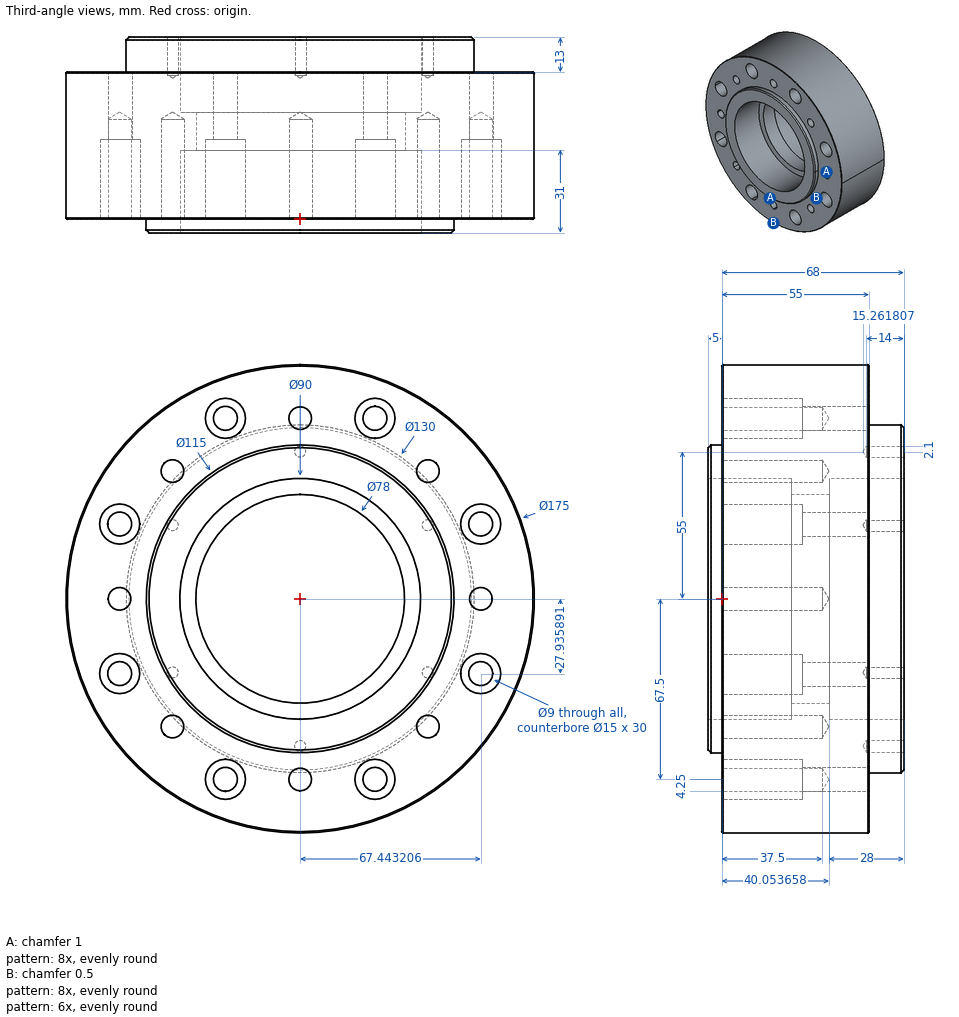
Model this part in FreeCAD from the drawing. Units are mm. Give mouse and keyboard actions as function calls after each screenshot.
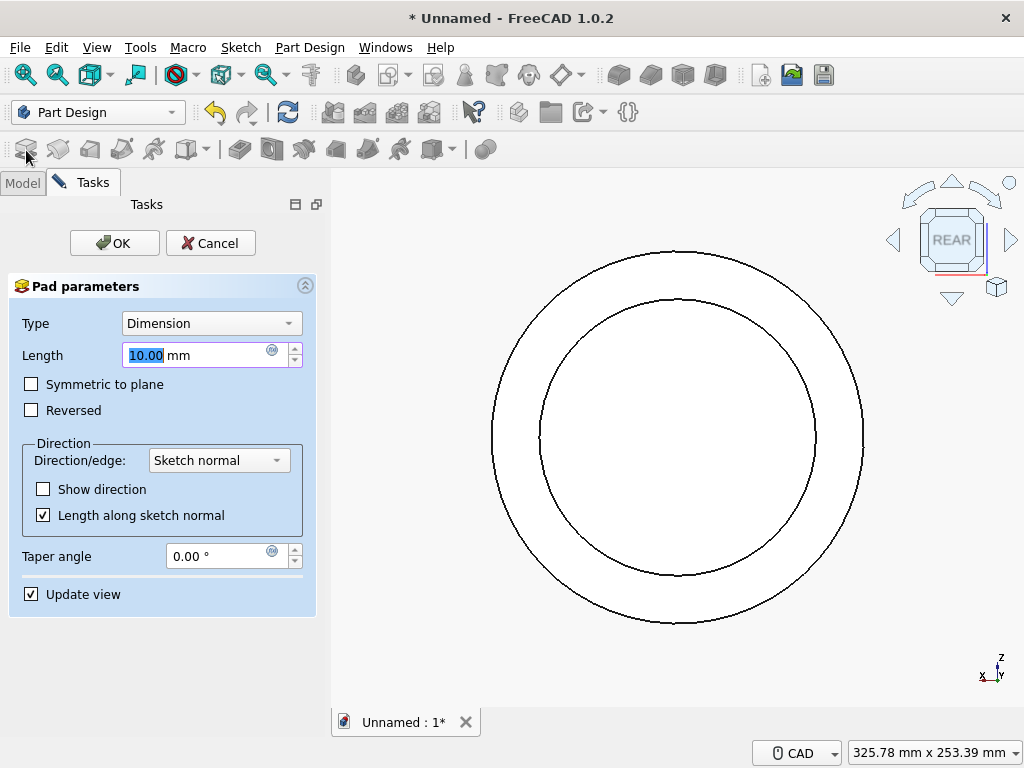
text(5)
key(Tab)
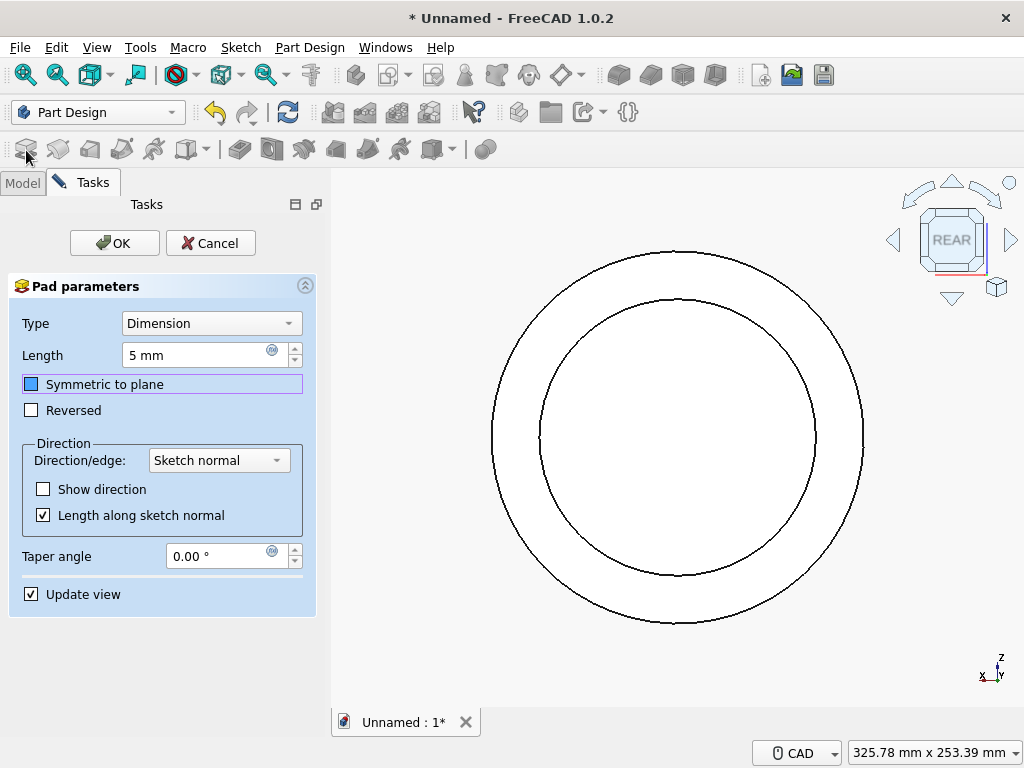
click(115, 243)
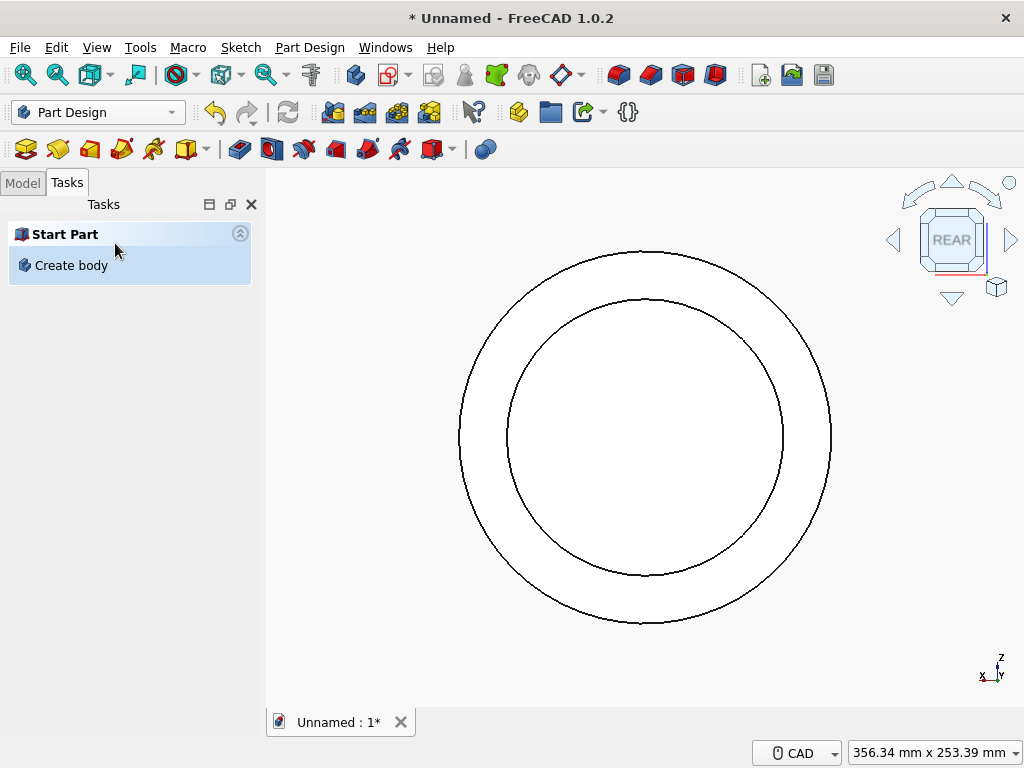
key(0)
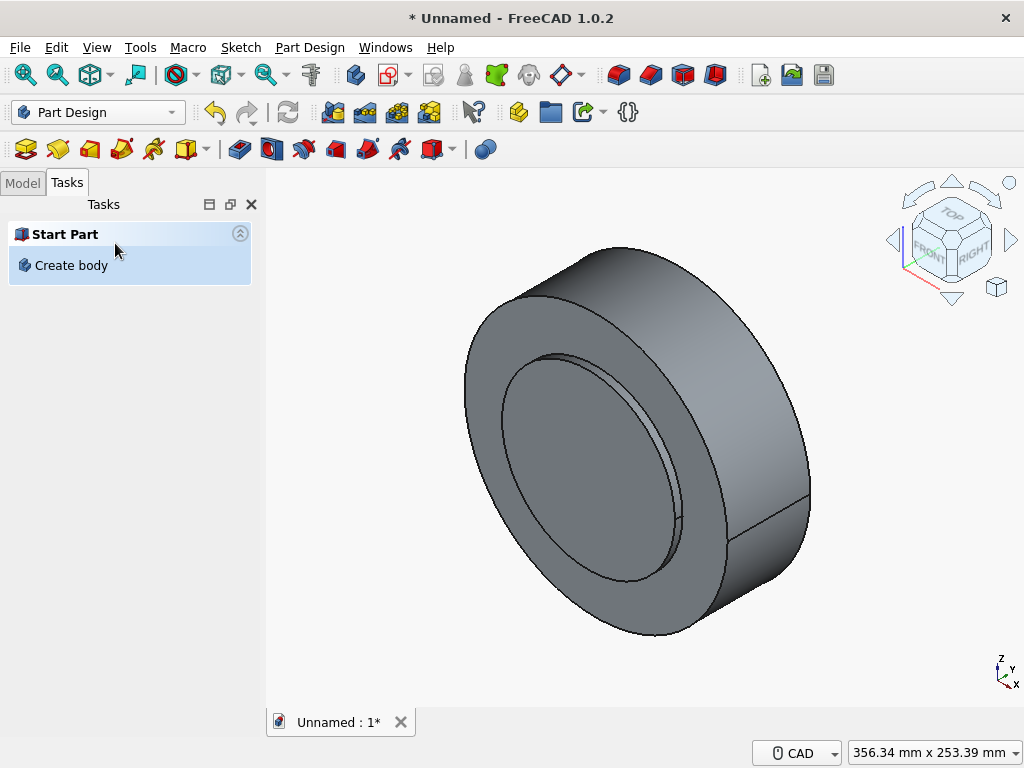
click(588, 469)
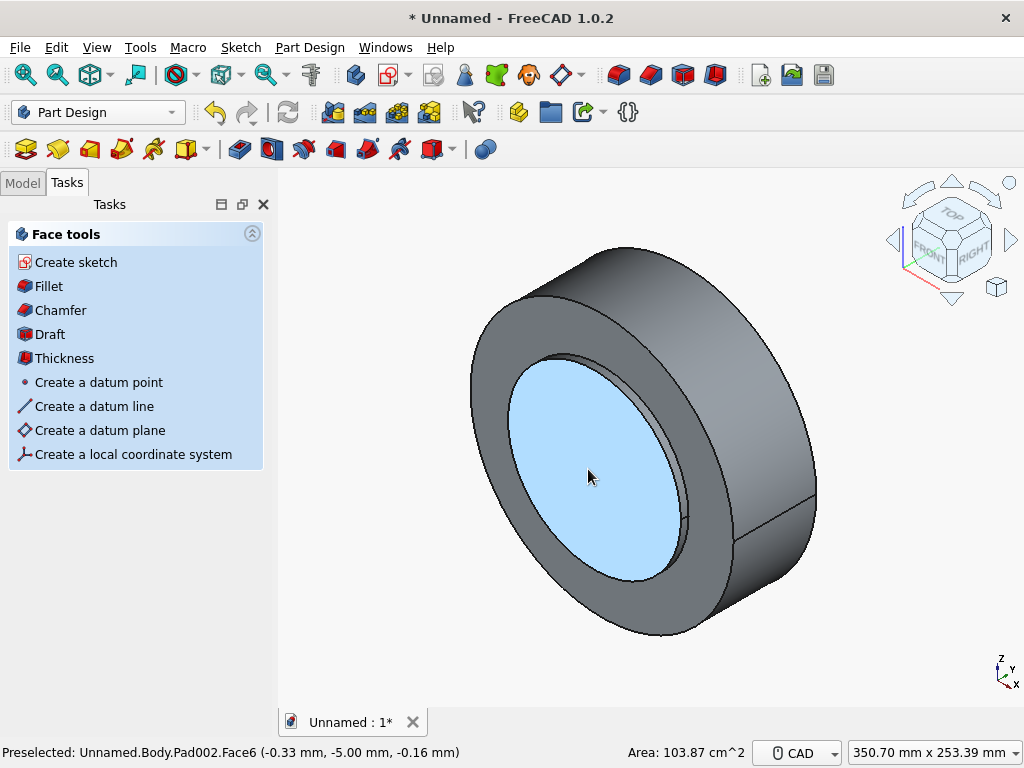
click(388, 76)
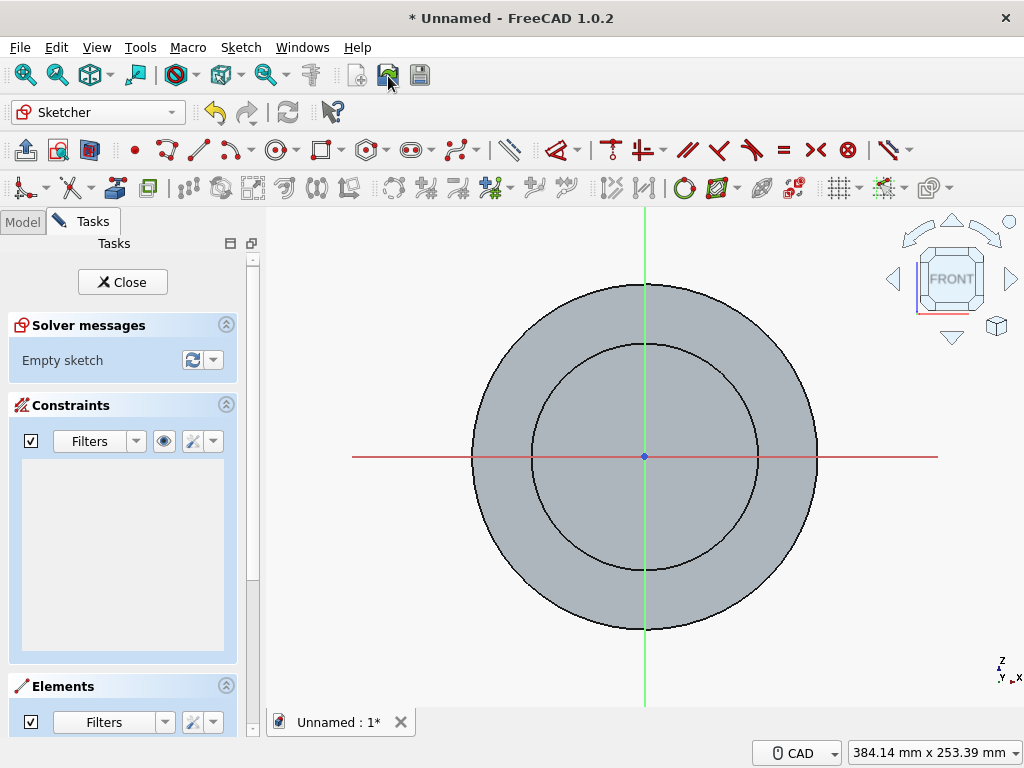
scroll(728, 457, up, 3)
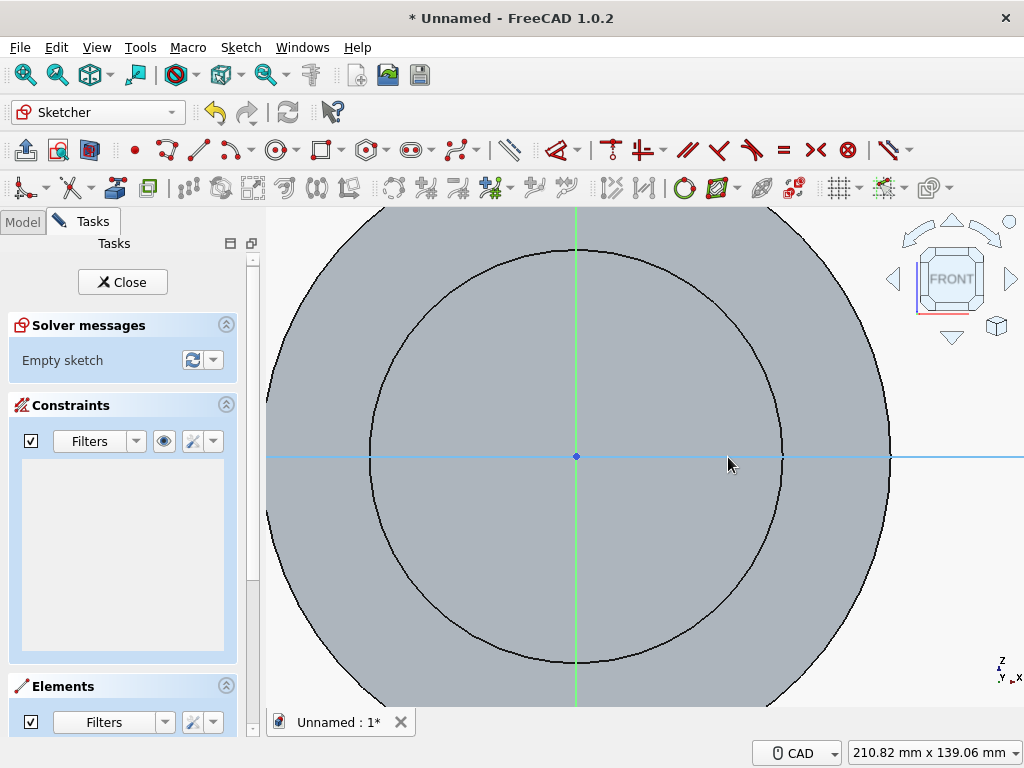
click(276, 150)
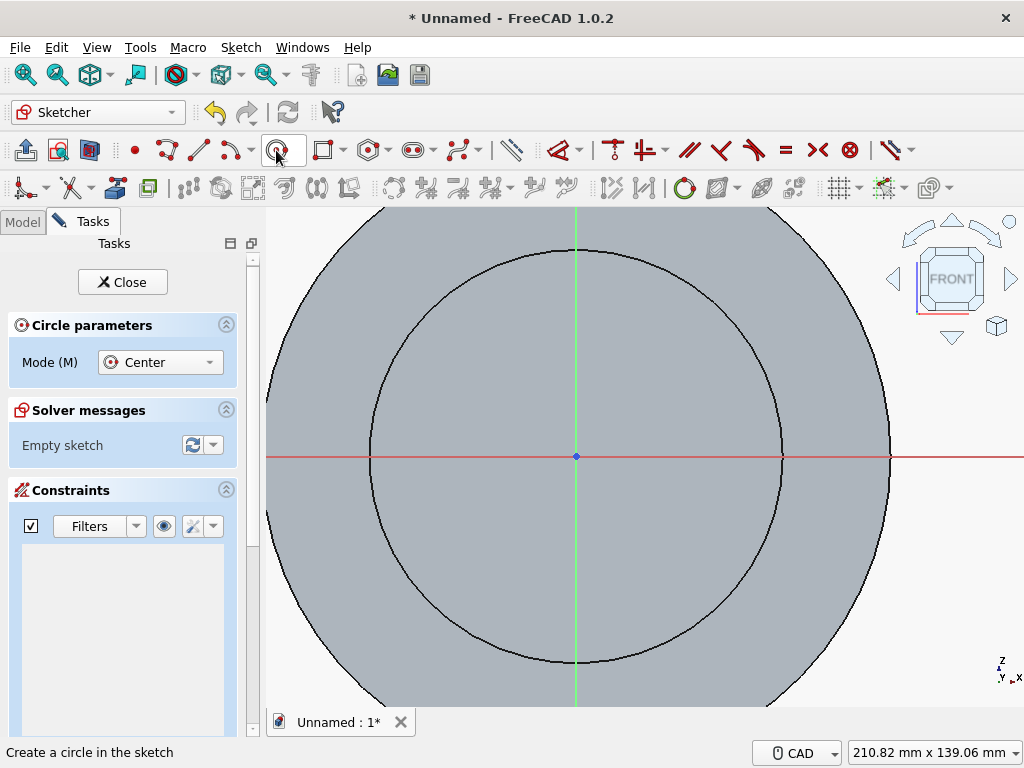
click(576, 457)
click(690, 342)
key(Escape)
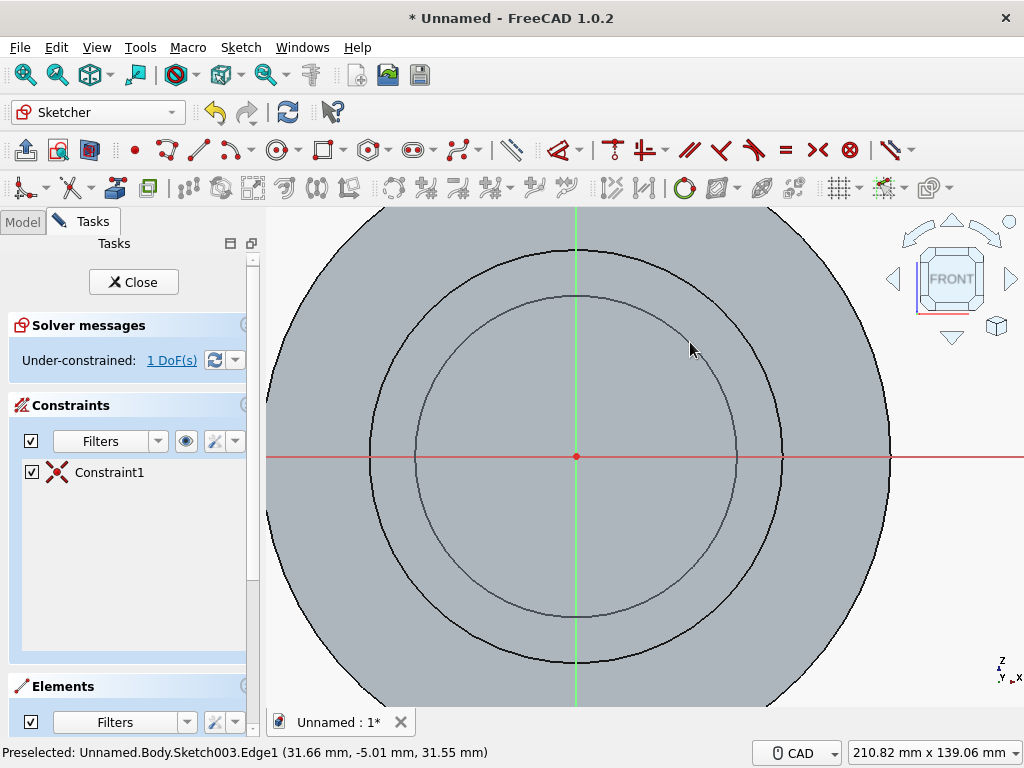
click(558, 150)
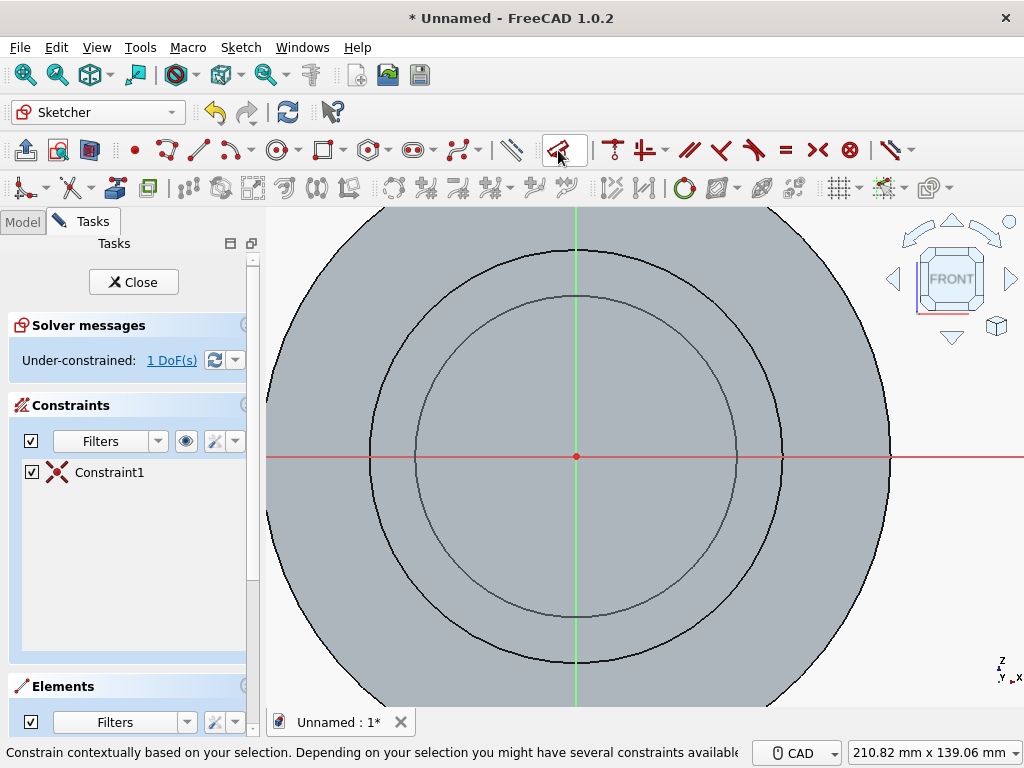
click(689, 342)
click(711, 319)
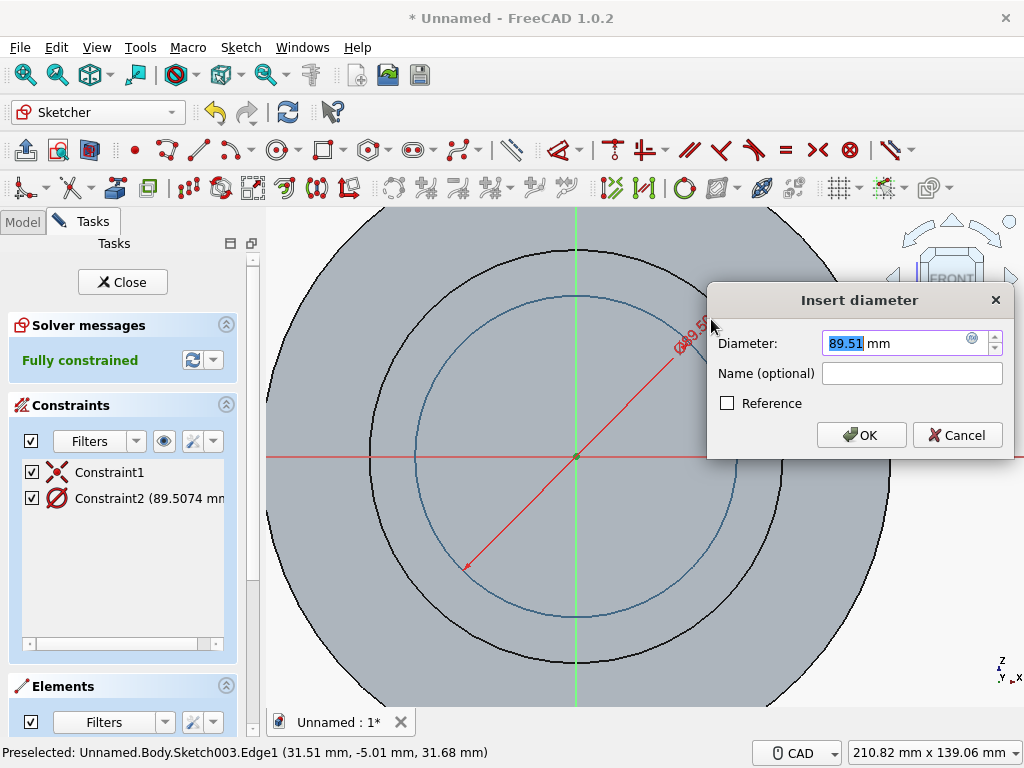
text(90)
key(Return)
key(Escape)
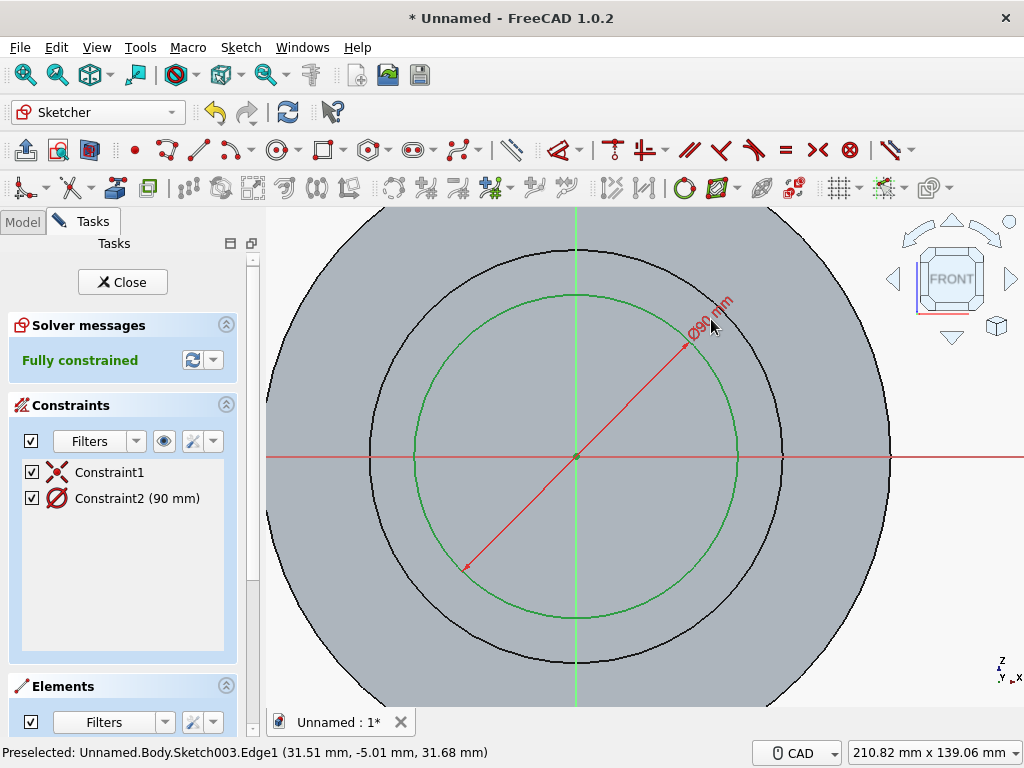
click(123, 282)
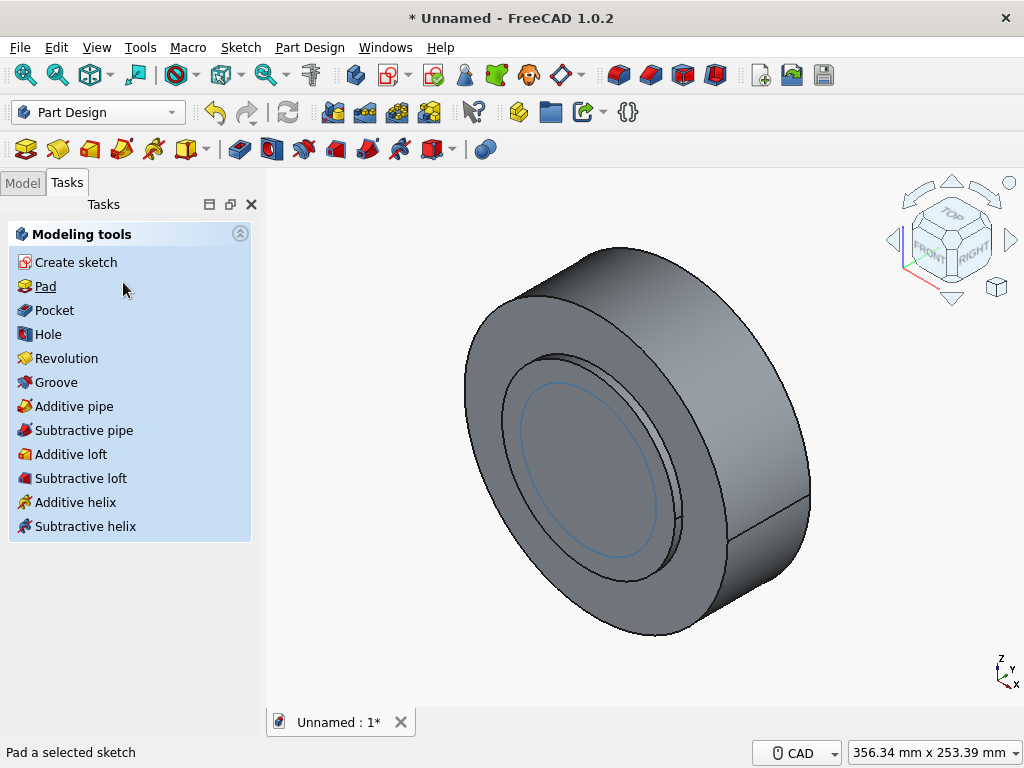
click(240, 150)